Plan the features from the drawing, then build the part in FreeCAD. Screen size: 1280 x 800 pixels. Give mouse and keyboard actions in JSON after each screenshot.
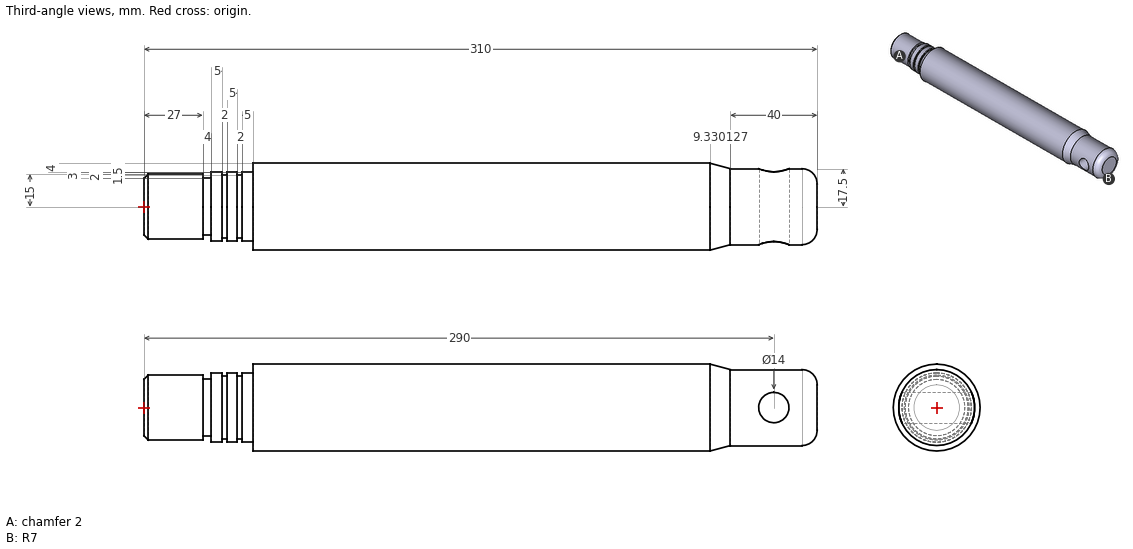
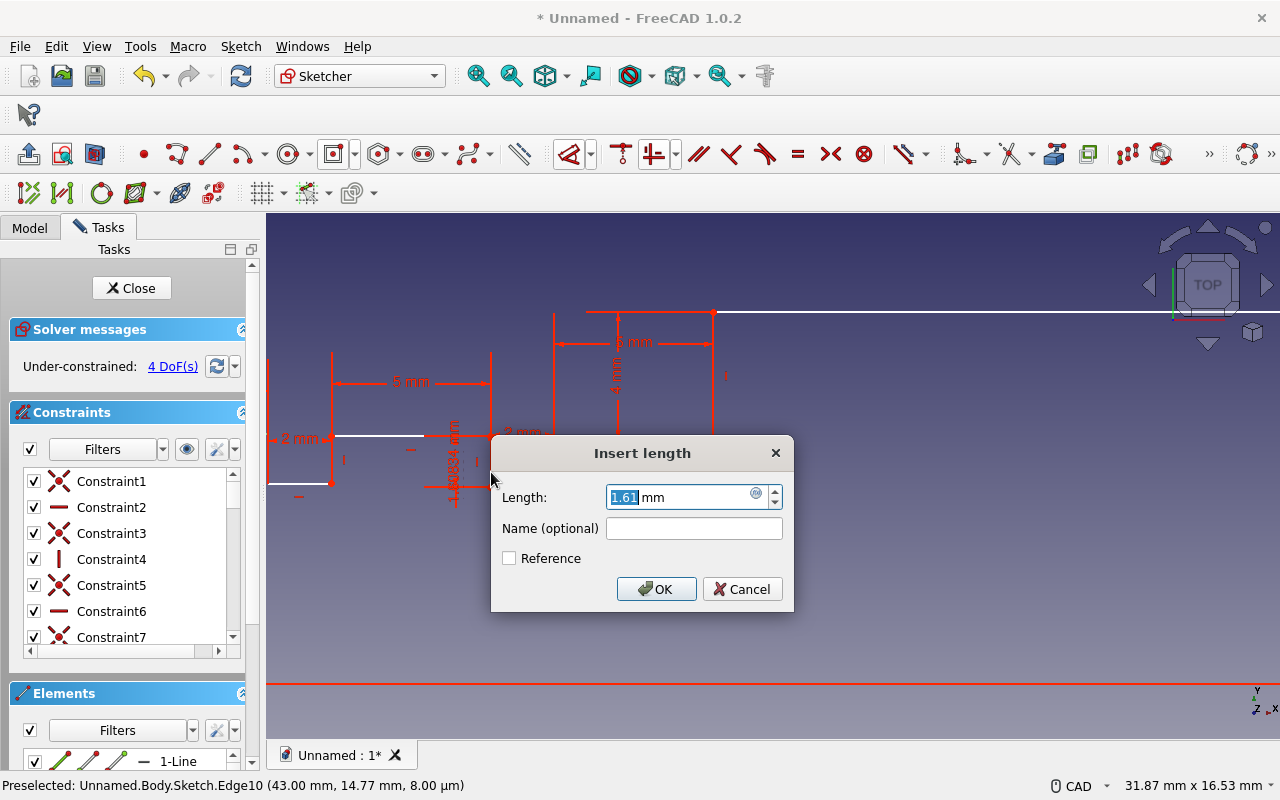
{"action": "type", "text": "1.5"}
{"action": "key", "text": "Return"}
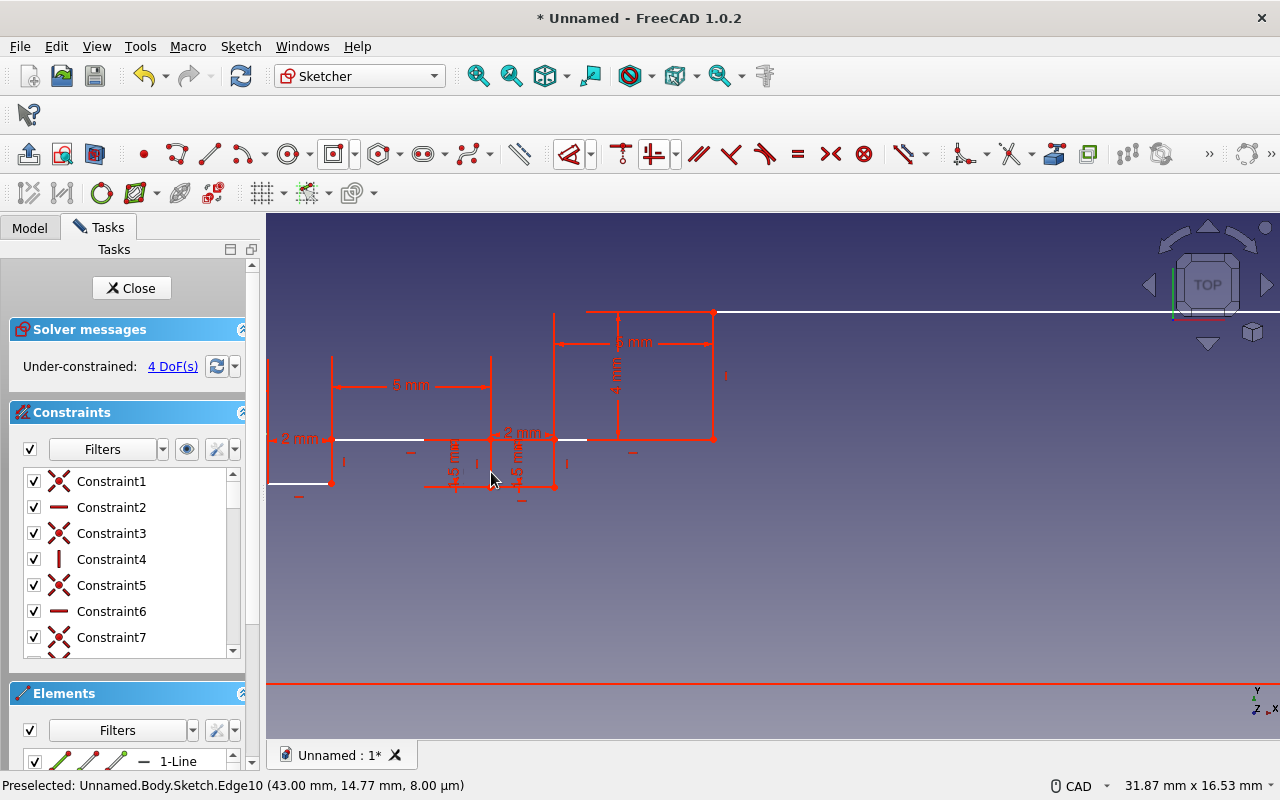
{"action": "left_click", "coordinate": [332, 453]}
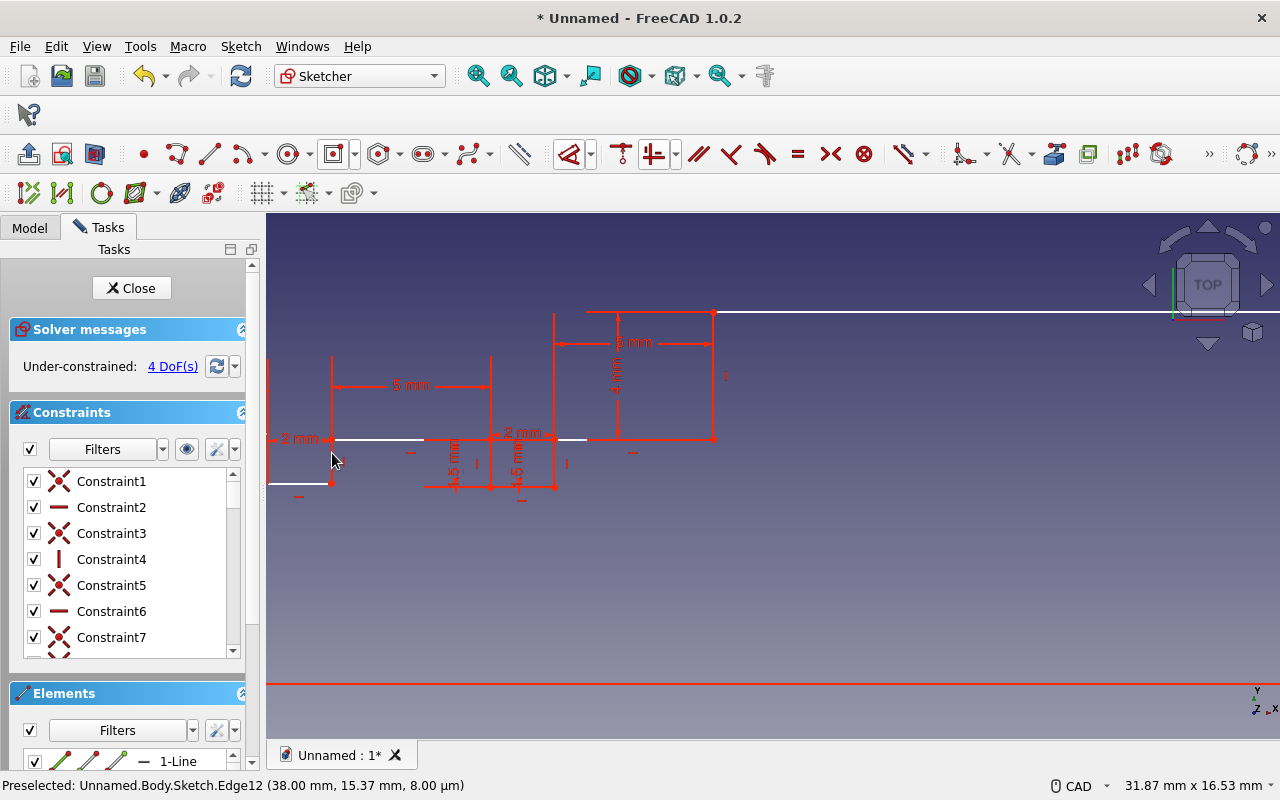
{"action": "left_click", "coordinate": [590, 154]}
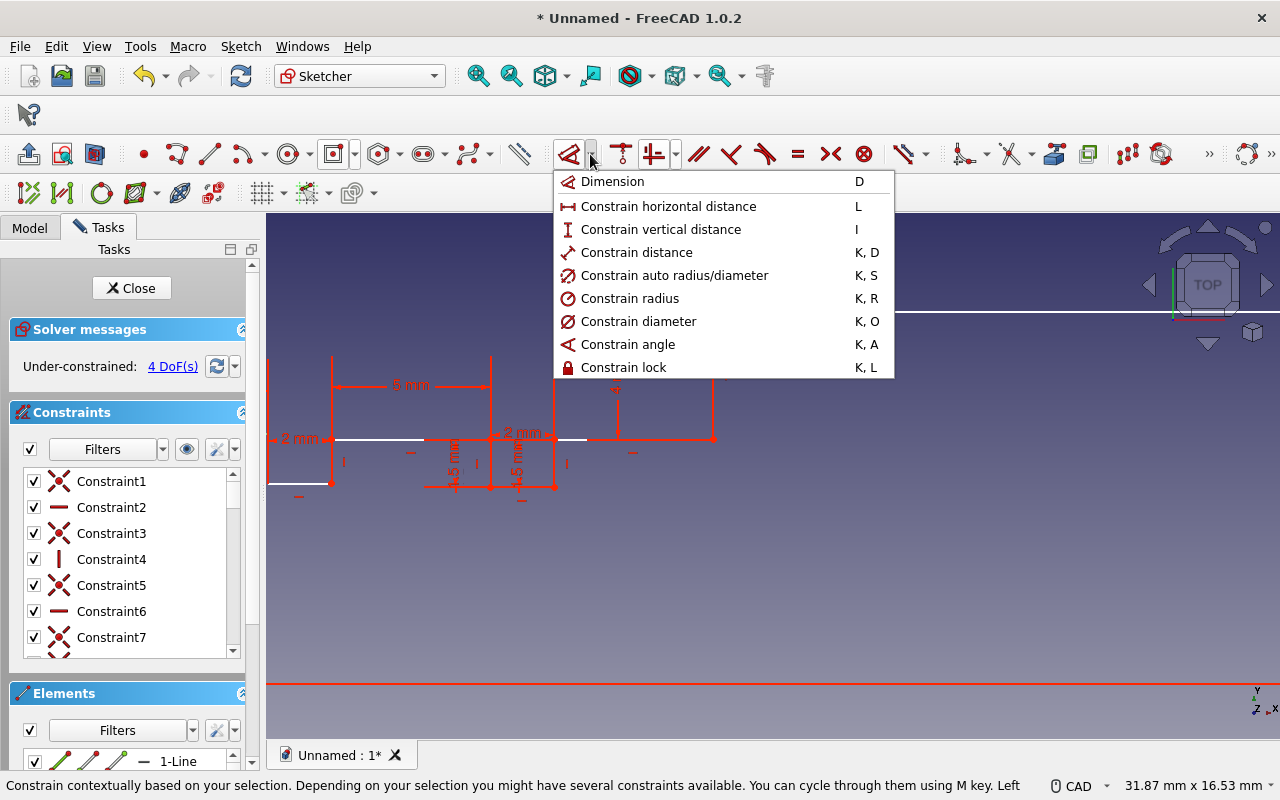
{"action": "left_click", "coordinate": [724, 230]}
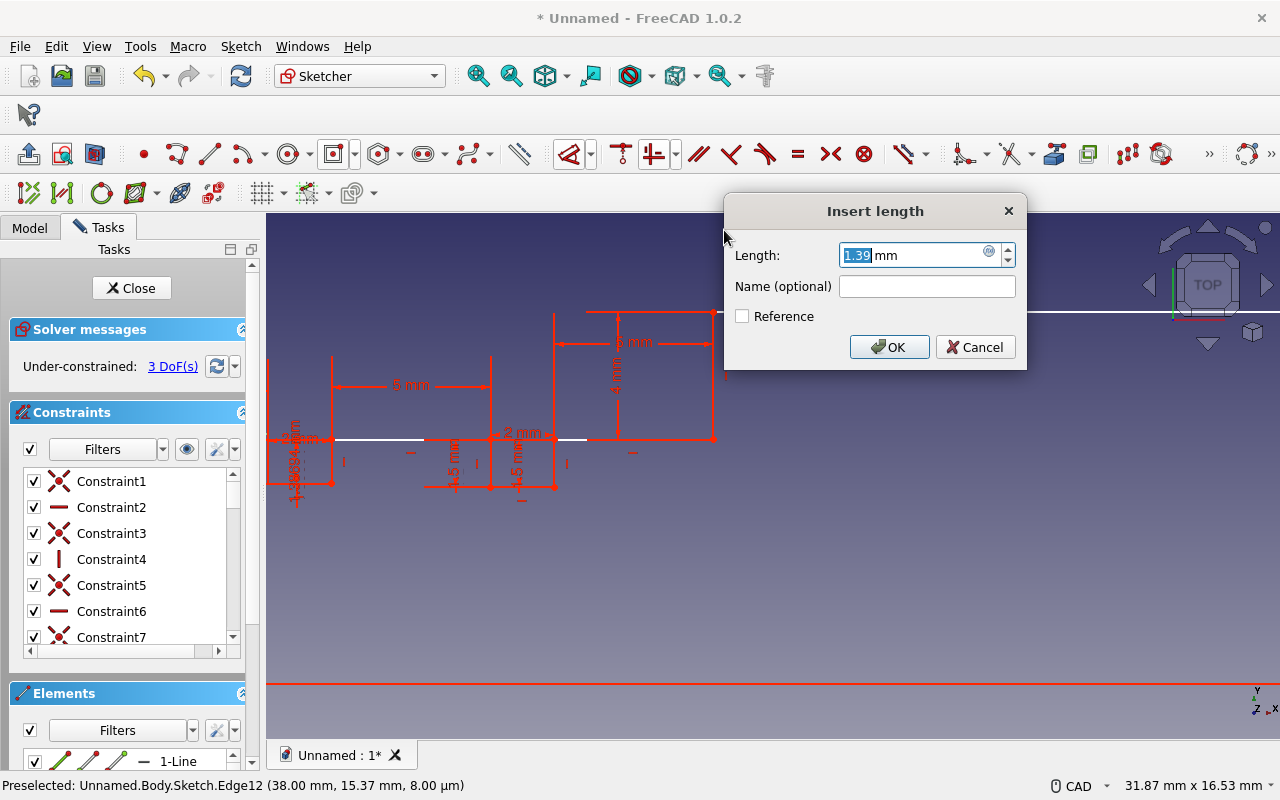
{"action": "type", "text": "1.5"}
{"action": "key", "text": "Return"}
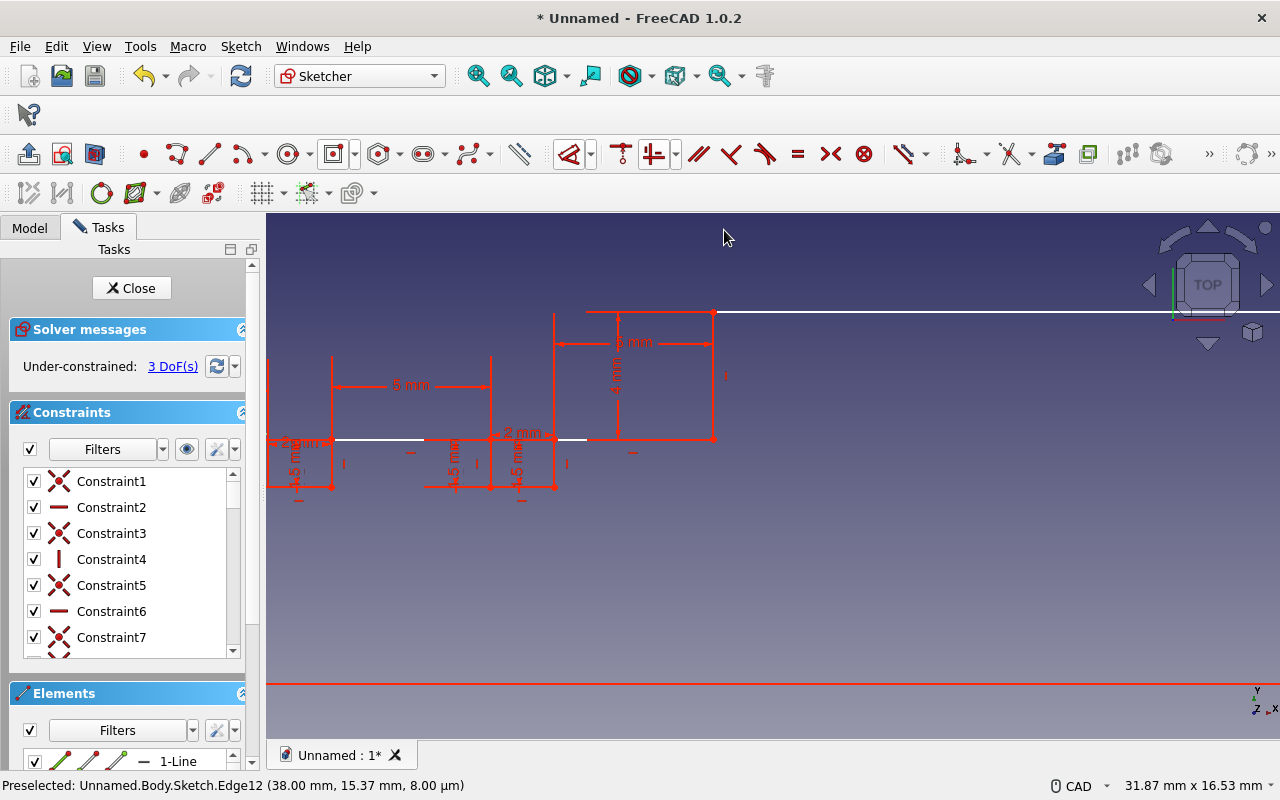
{"action": "scroll", "coordinate": [488, 466], "scroll_direction": "down", "scroll_amount": 14}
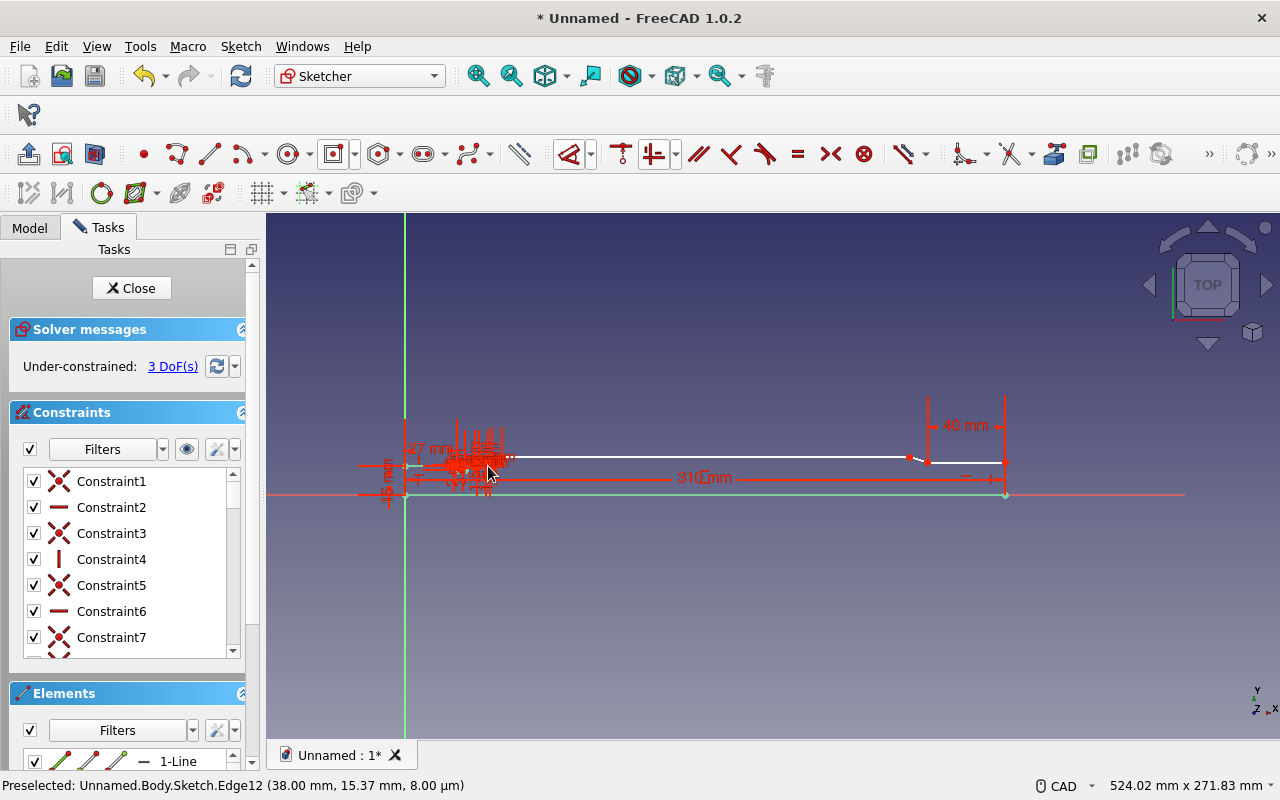
{"action": "scroll", "coordinate": [475, 467], "scroll_direction": "up", "scroll_amount": 14}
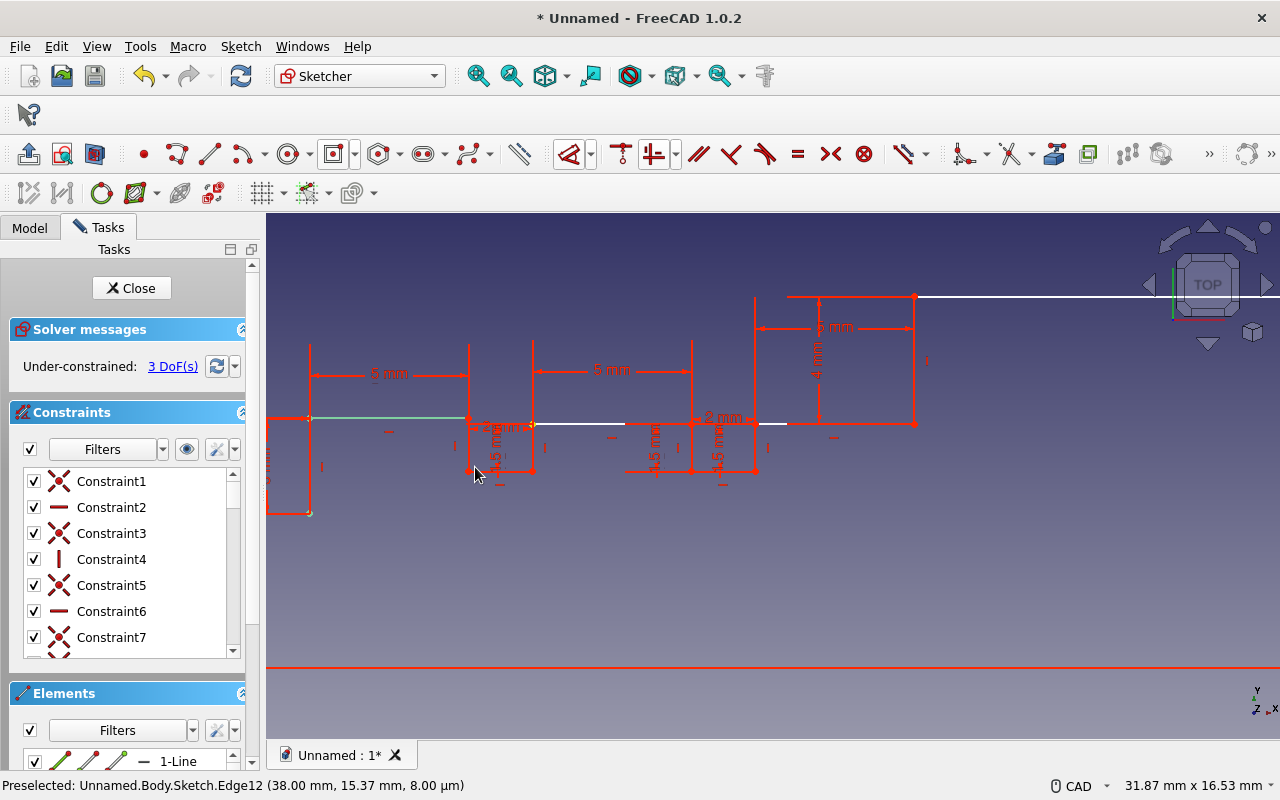
{"action": "left_click", "coordinate": [469, 456]}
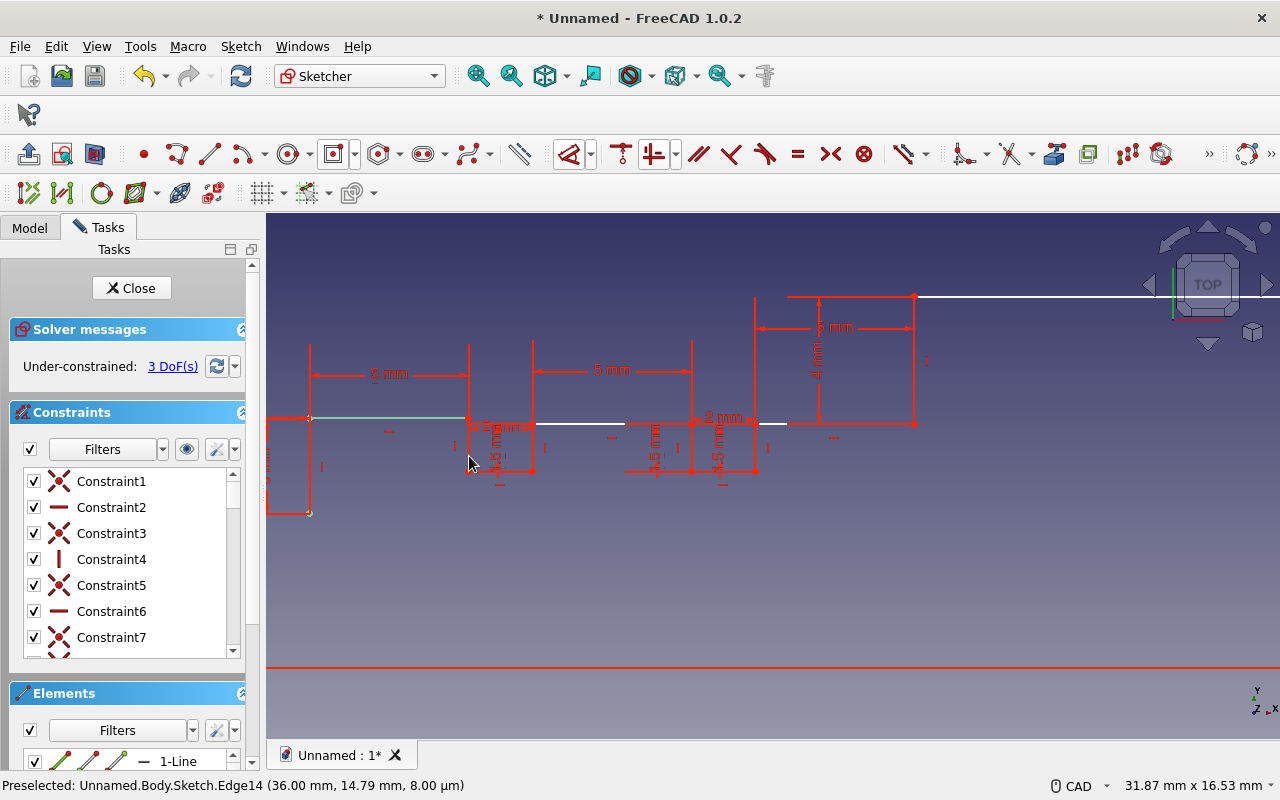
{"action": "key", "text": "i"}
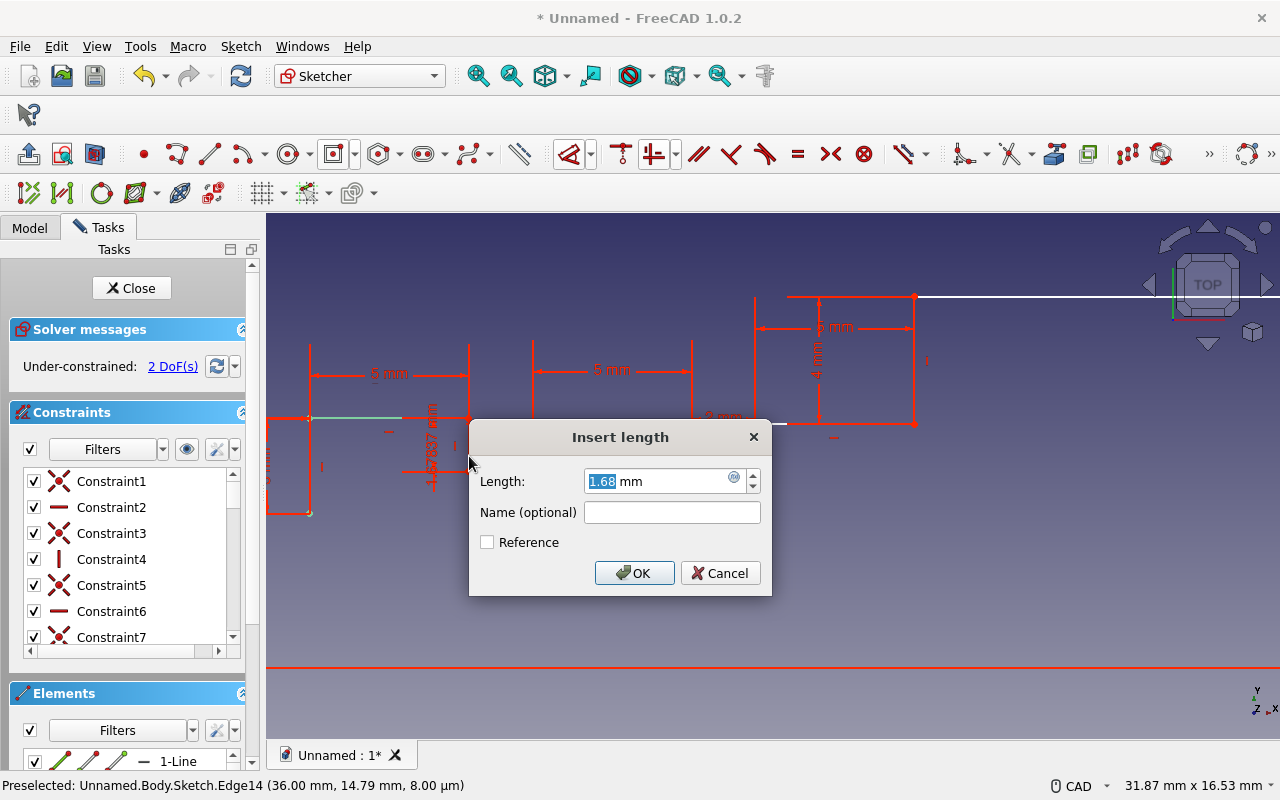
{"action": "type", "text": "1.5"}
{"action": "key", "text": "Return"}